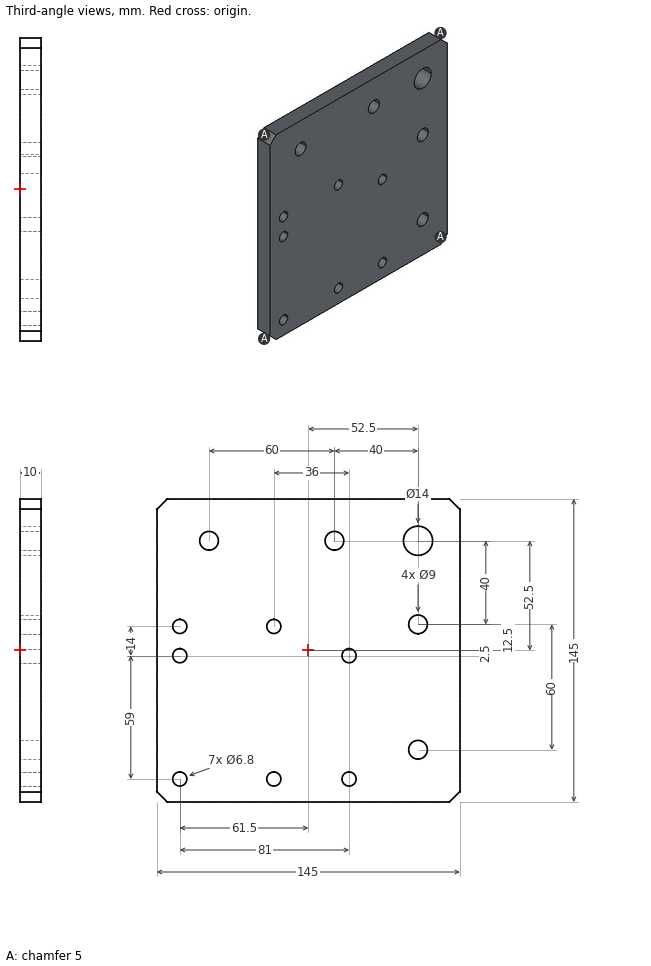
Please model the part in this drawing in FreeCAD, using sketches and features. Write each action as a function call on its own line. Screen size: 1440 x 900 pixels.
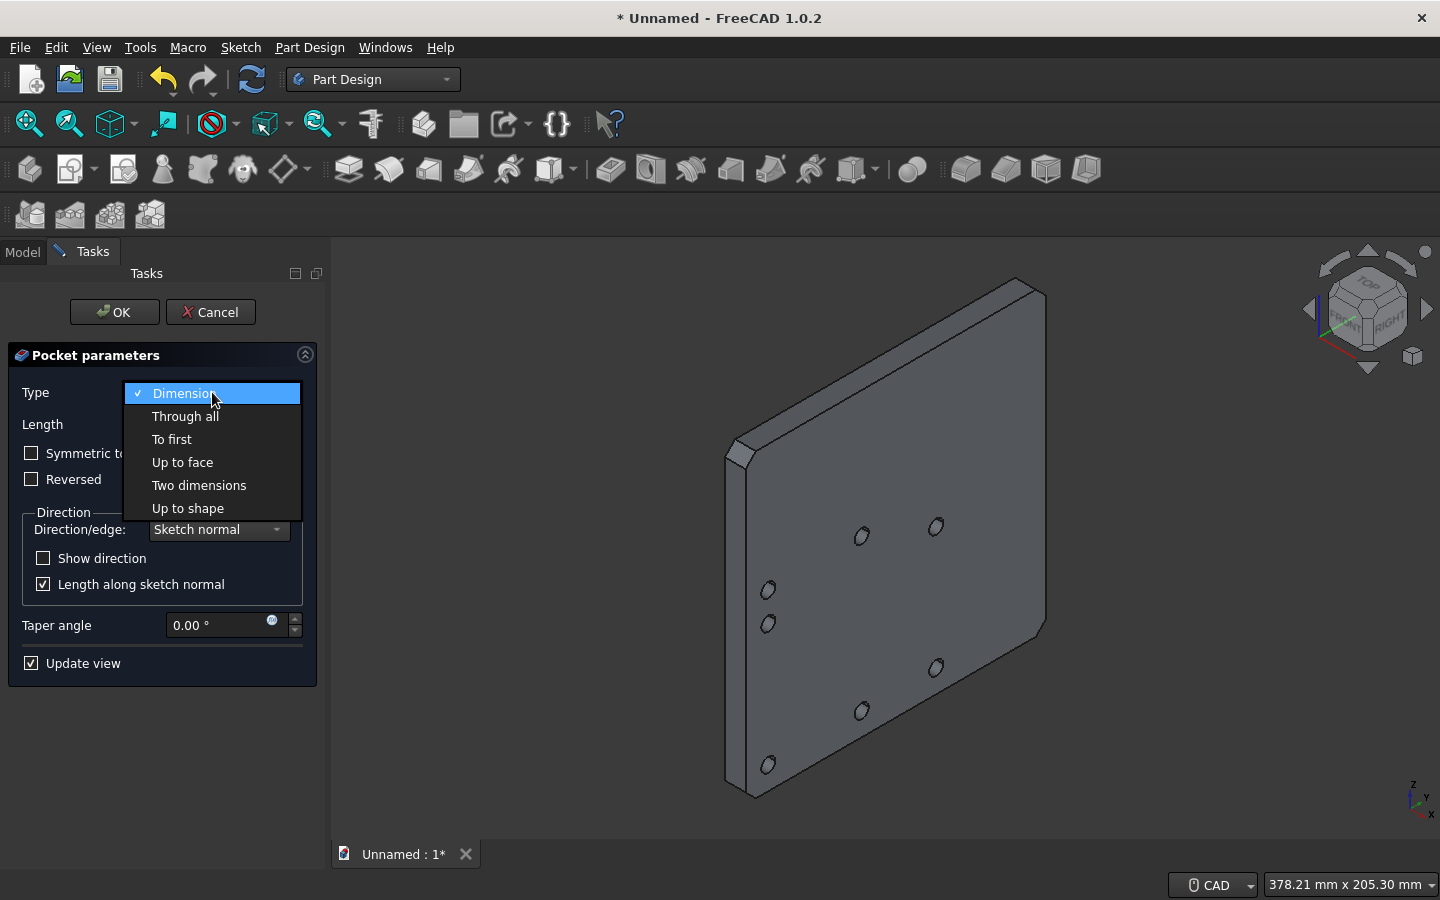
click(212, 416)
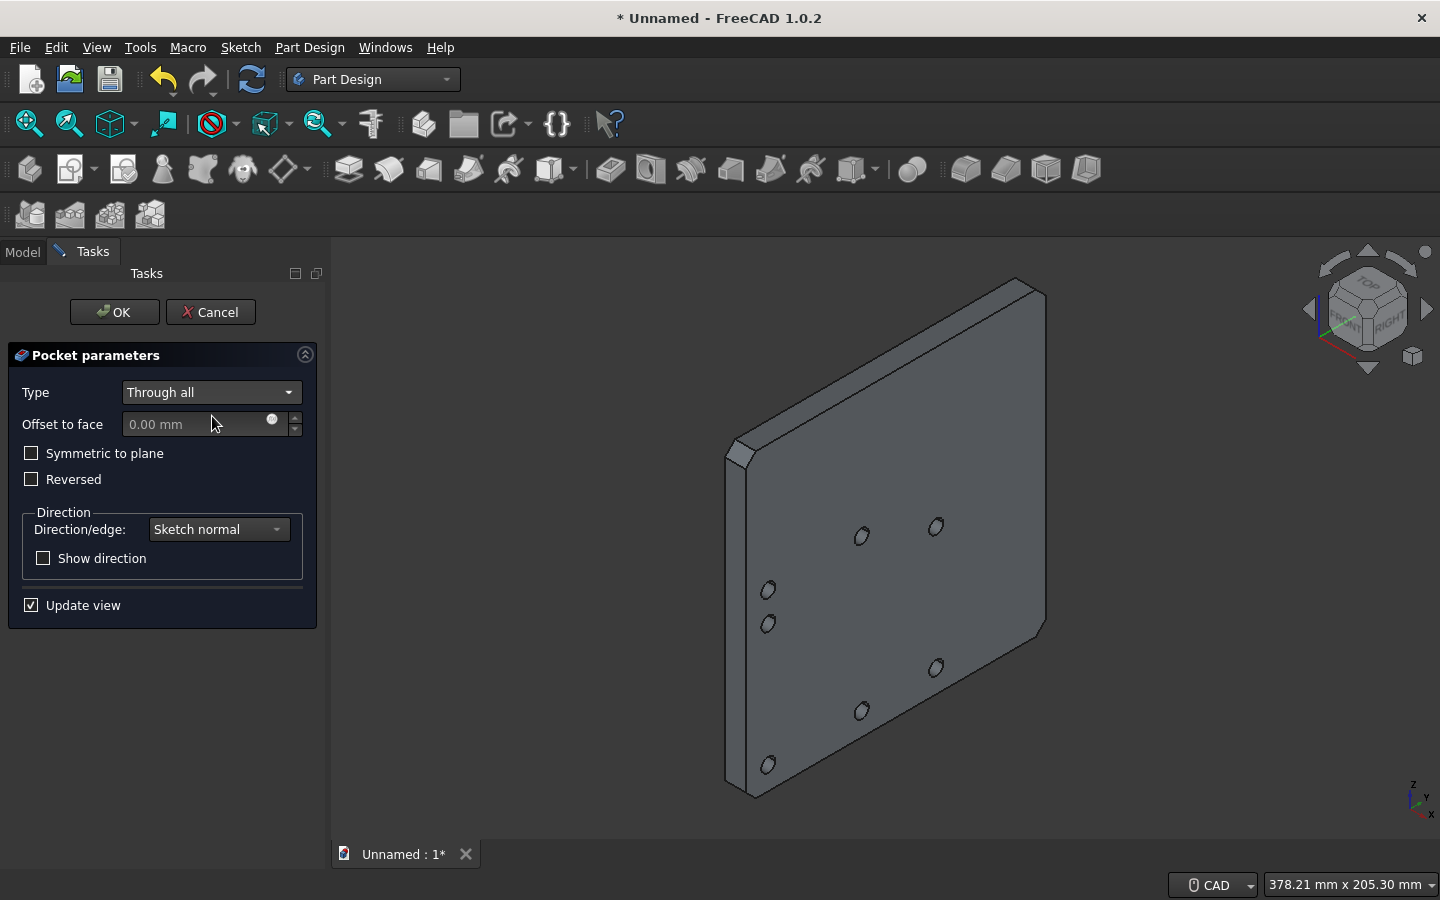
click(115, 312)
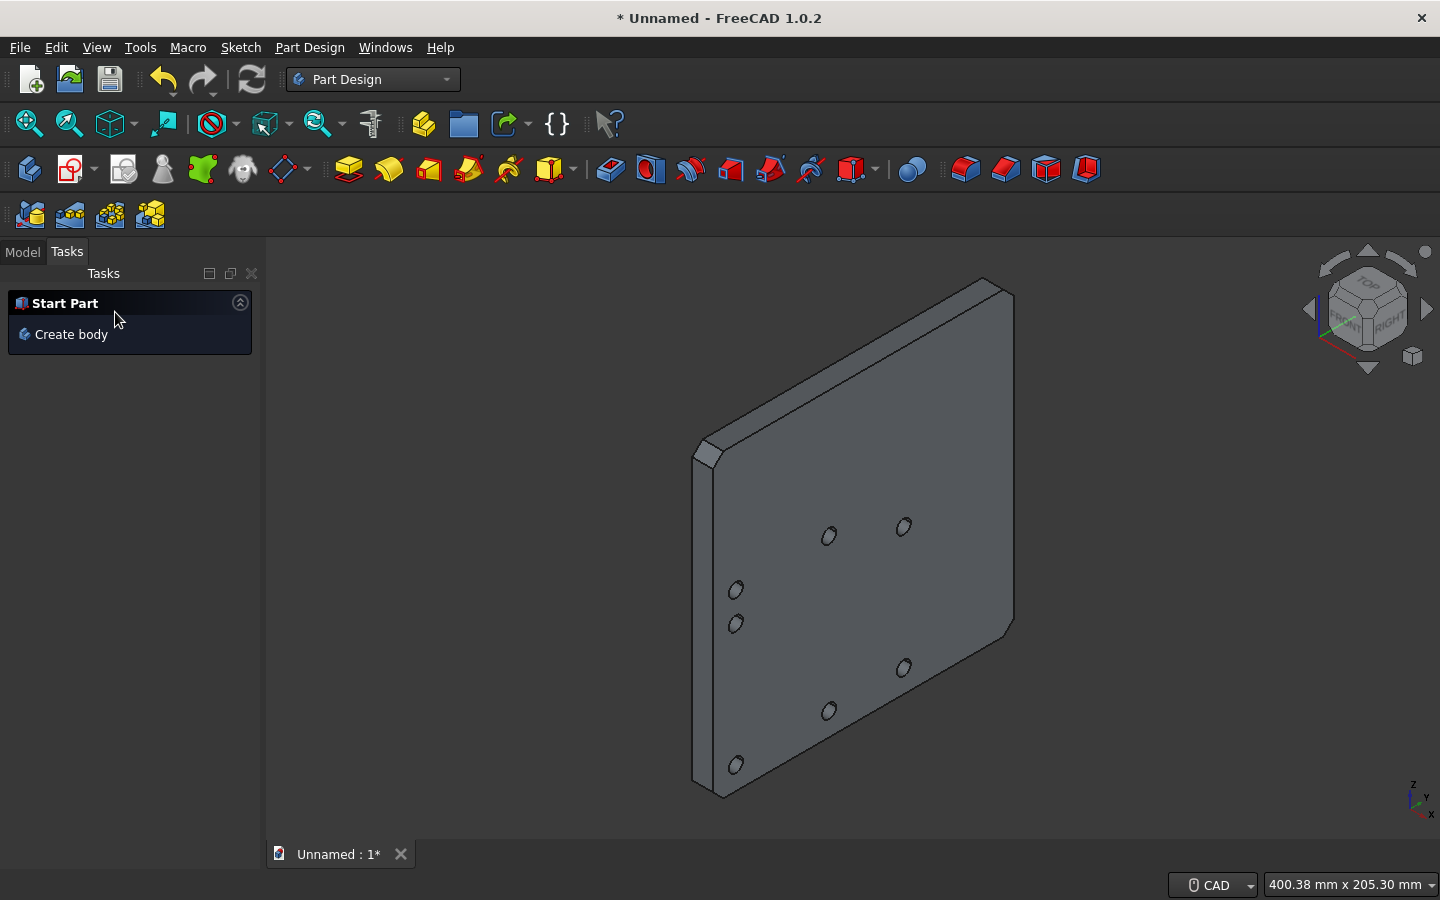
click(949, 394)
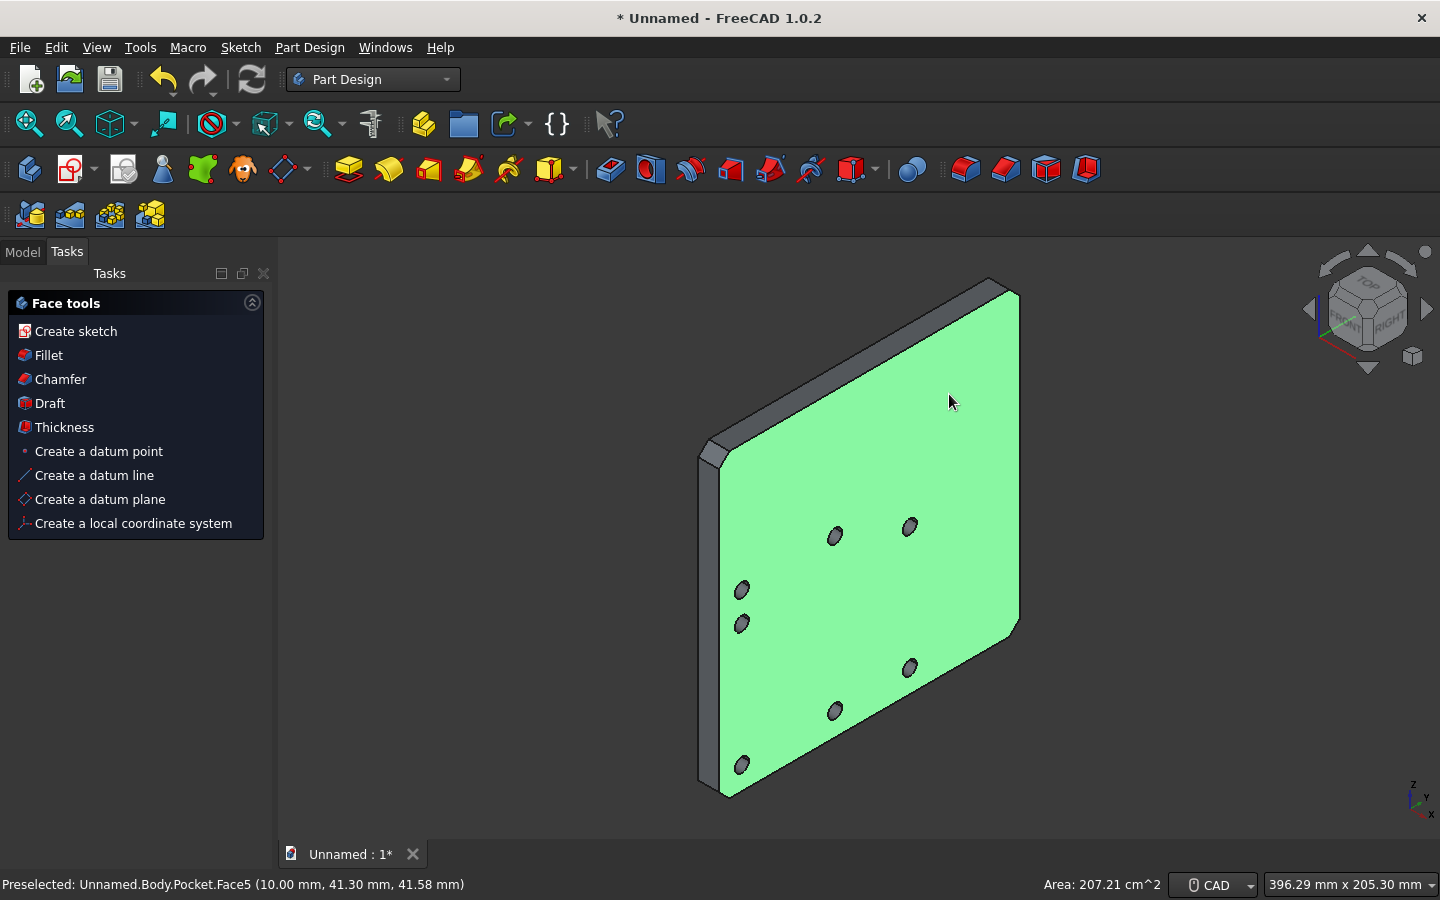
click(70, 170)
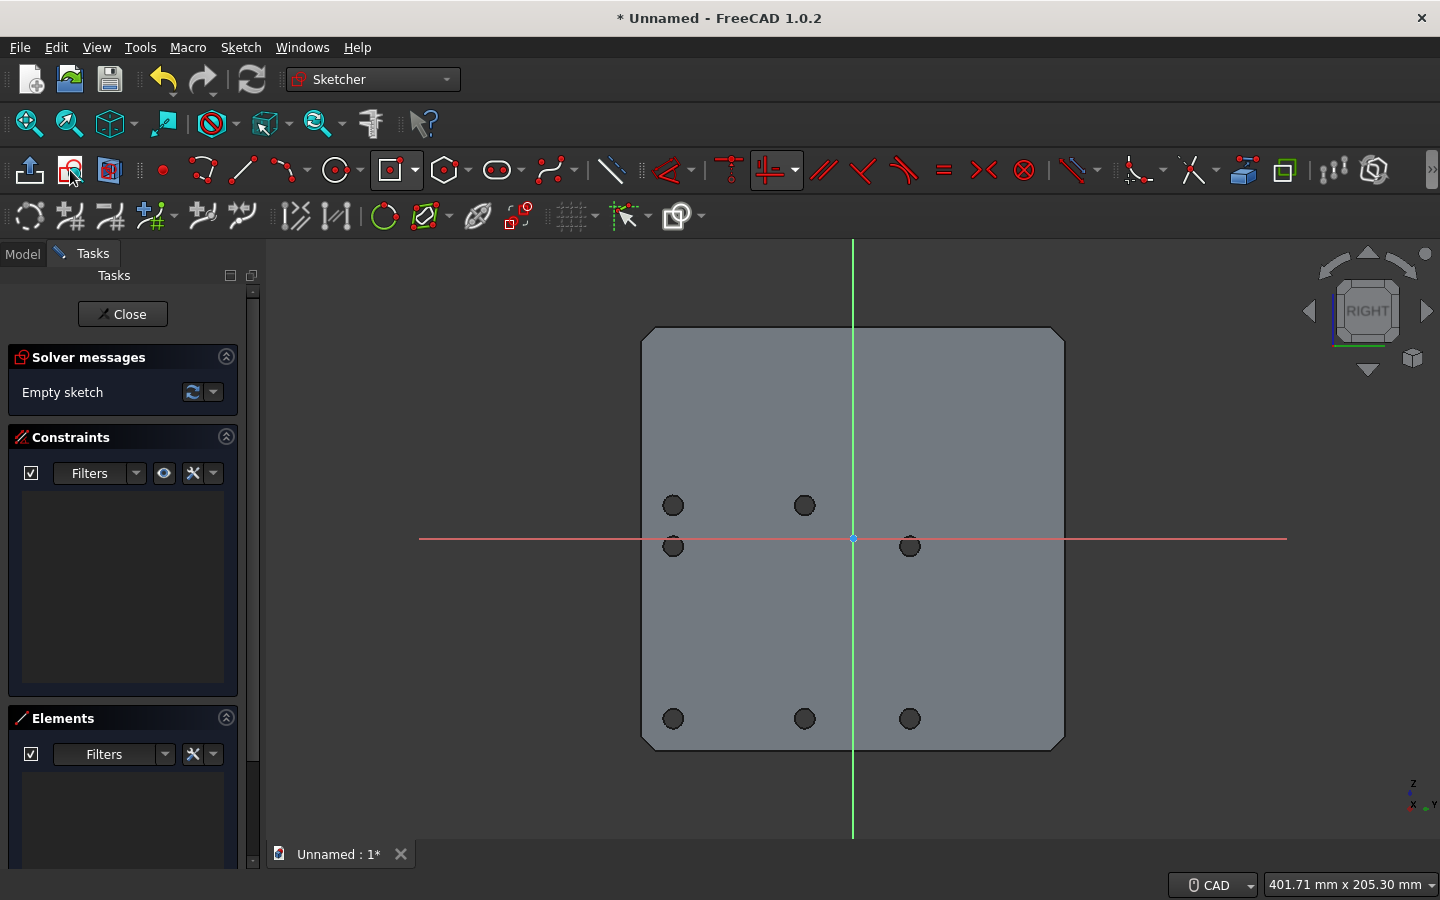
scroll(1034, 366, up, 11)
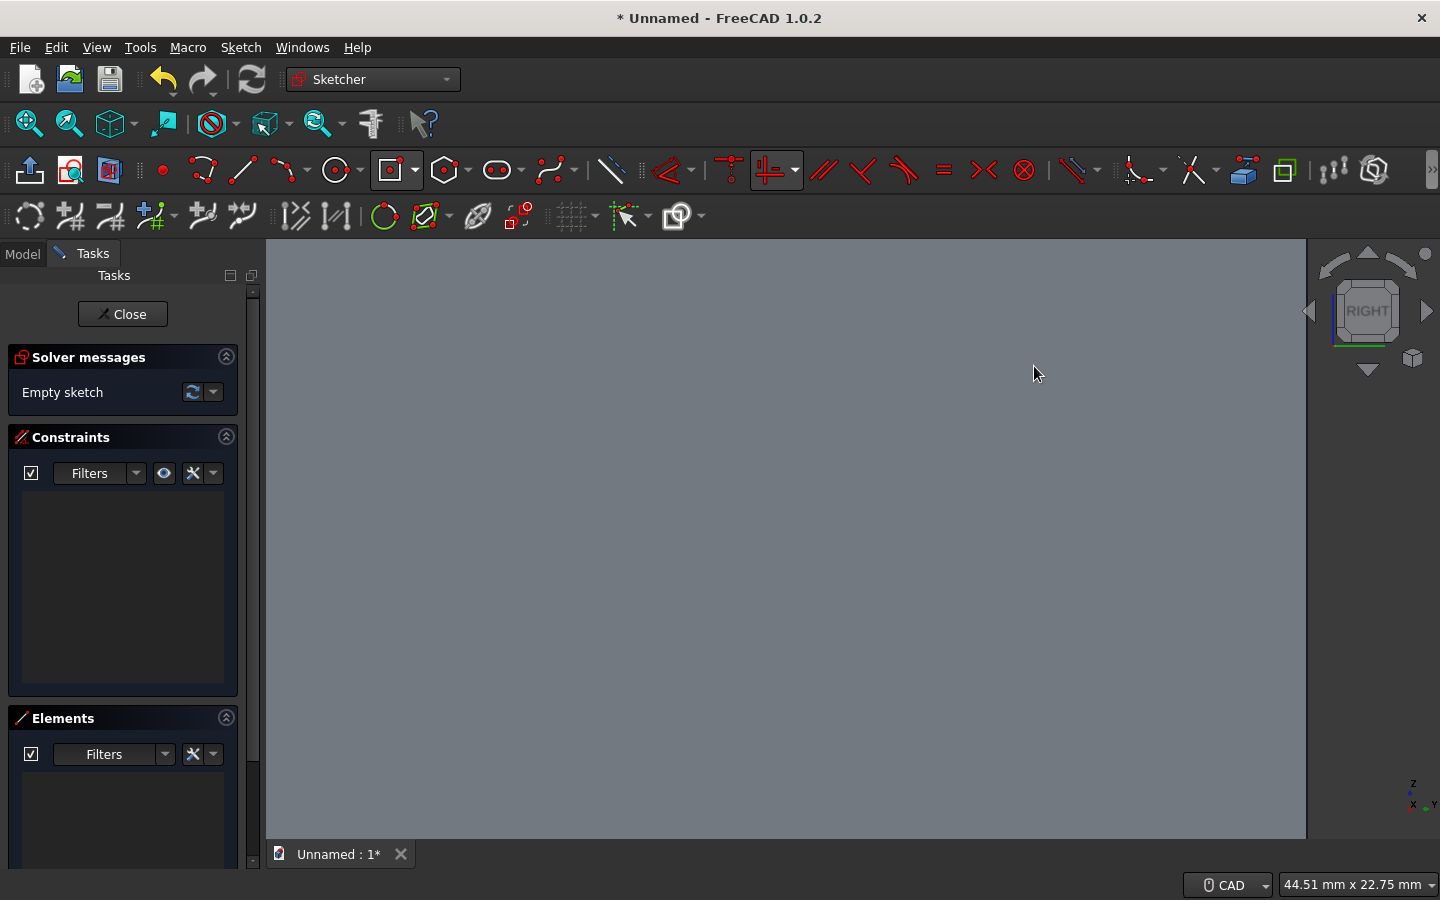
click(336, 170)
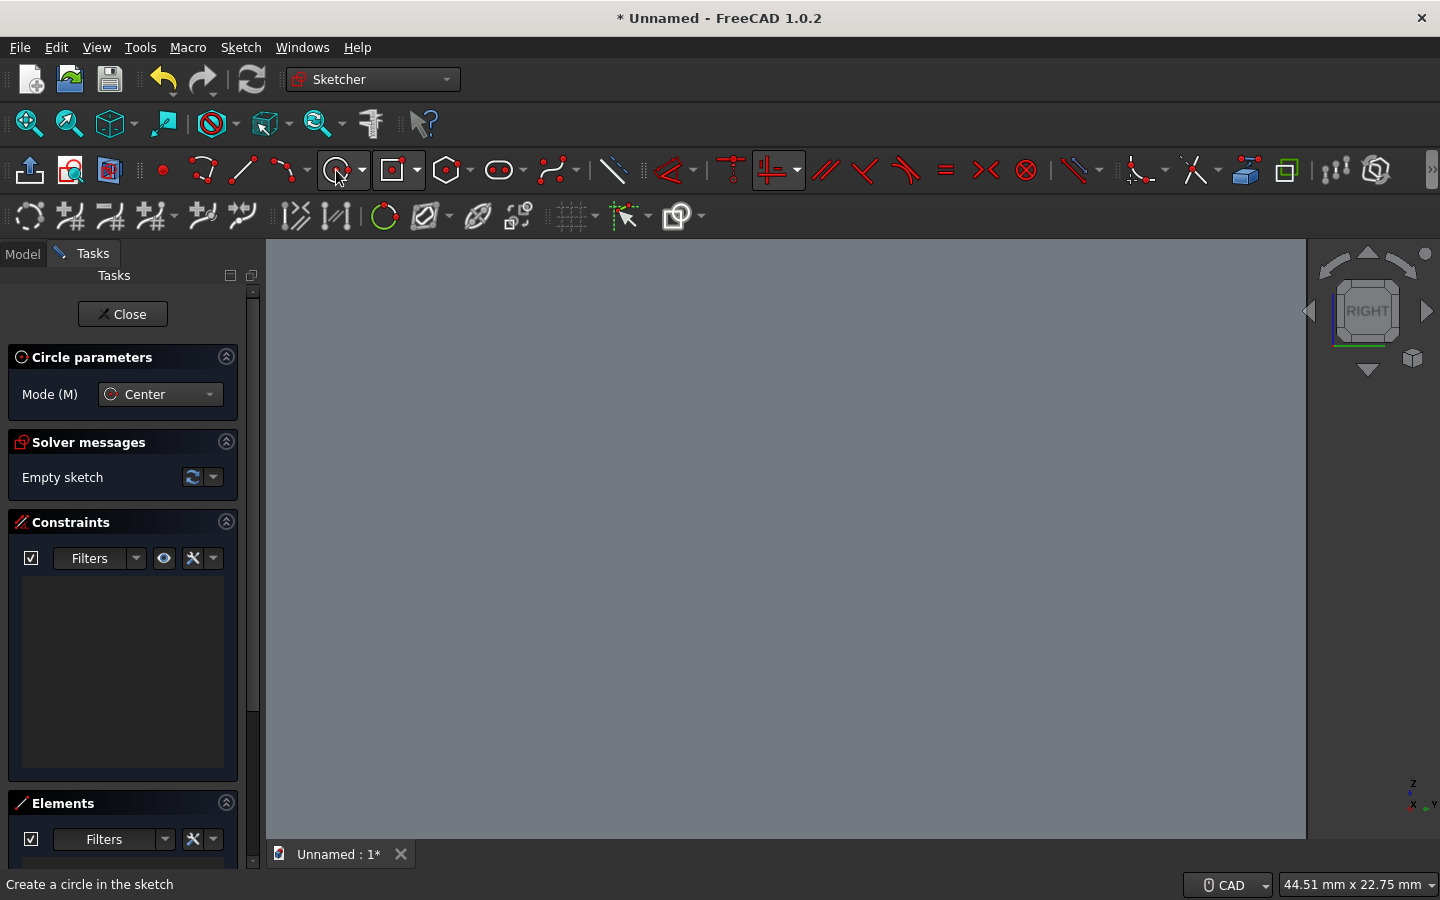
click(780, 541)
click(910, 410)
key(Escape)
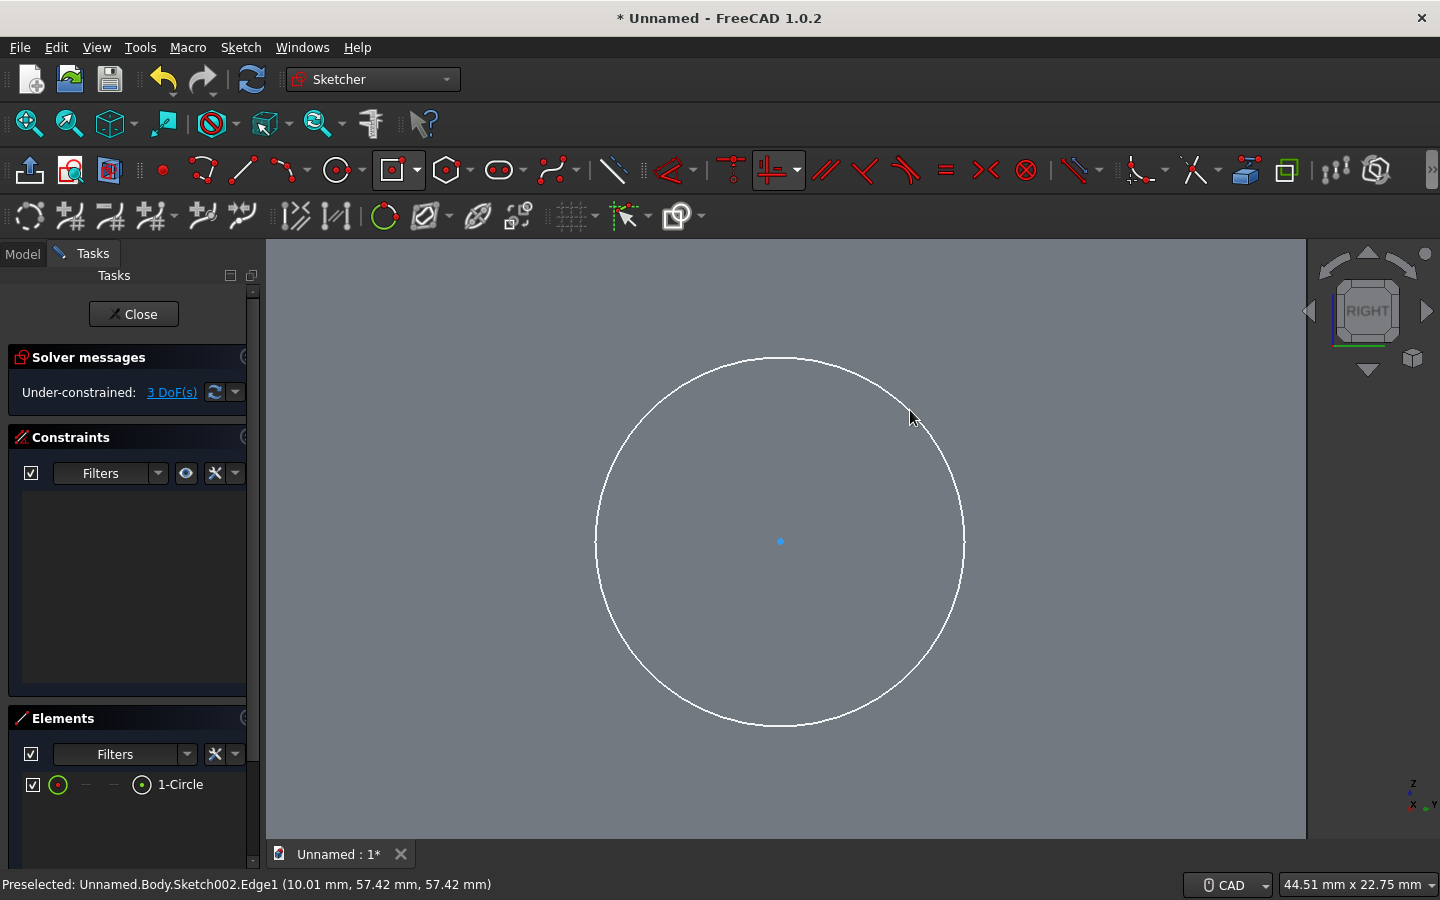
key(d)